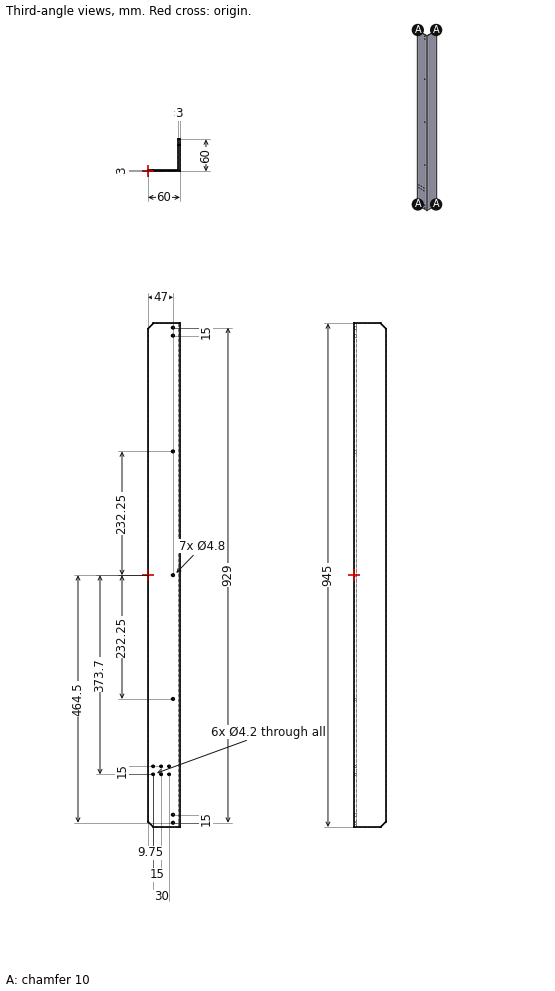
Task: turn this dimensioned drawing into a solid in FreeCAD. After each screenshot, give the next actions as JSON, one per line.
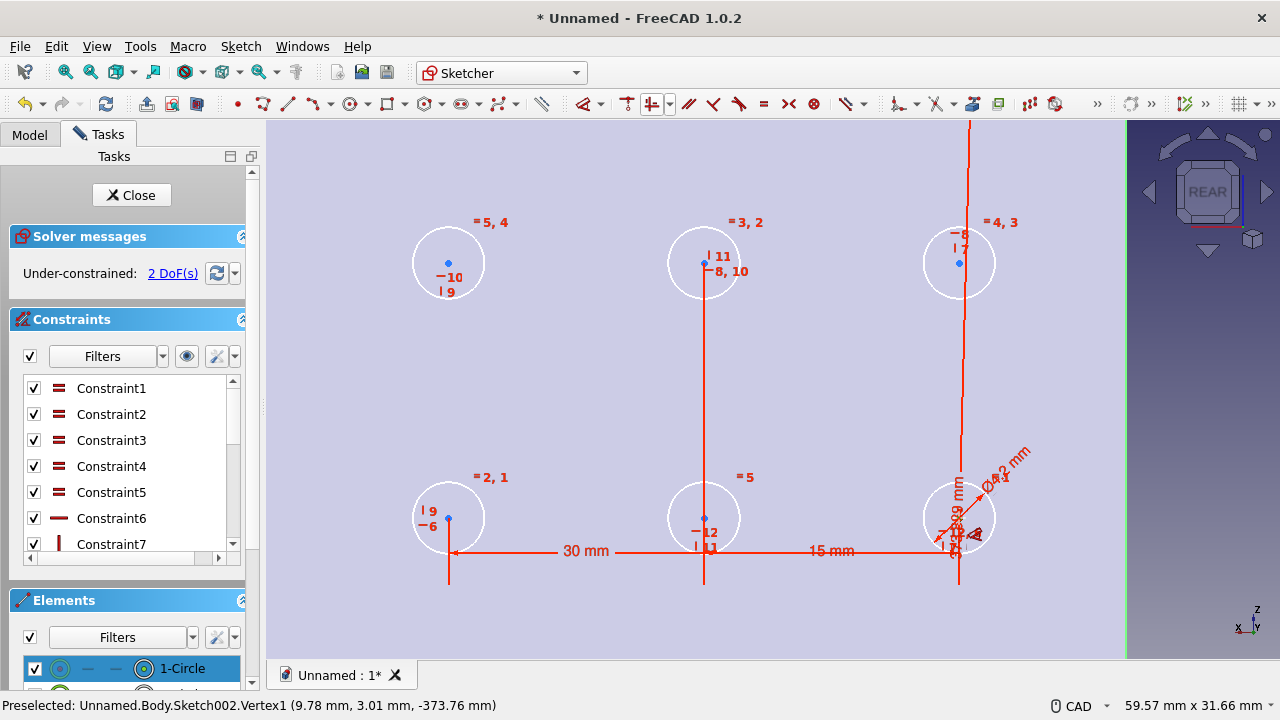
{"action": "left_click", "coordinate": [704, 263]}
{"action": "left_click", "coordinate": [993, 390]}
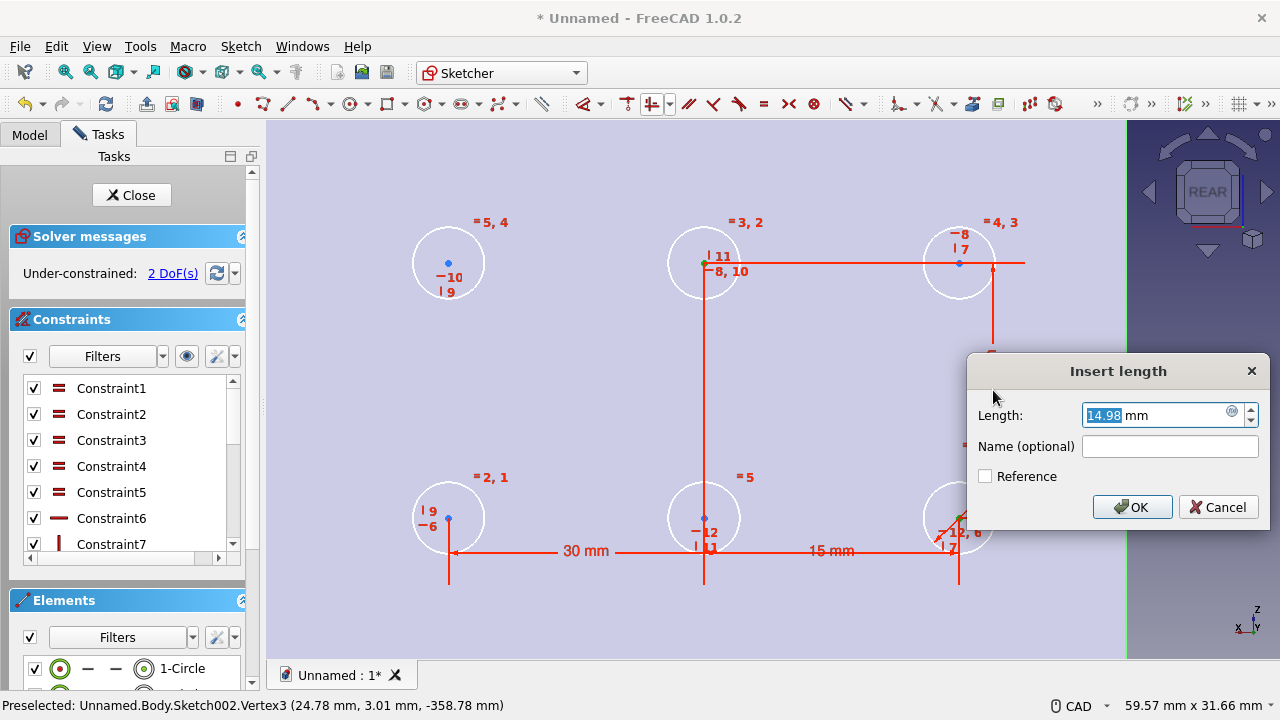
{"action": "type", "text": "15"}
{"action": "key", "text": "Return"}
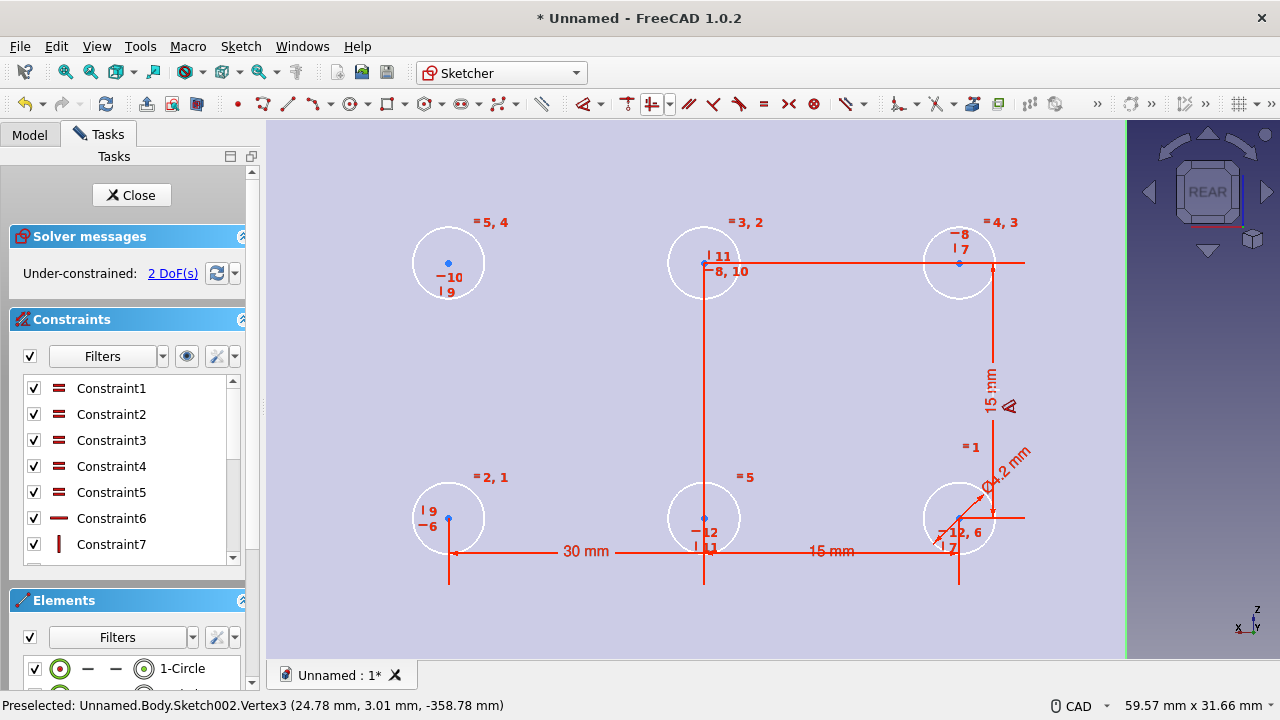
{"action": "left_click", "coordinate": [959, 518]}
{"action": "left_click", "coordinate": [1037, 552]}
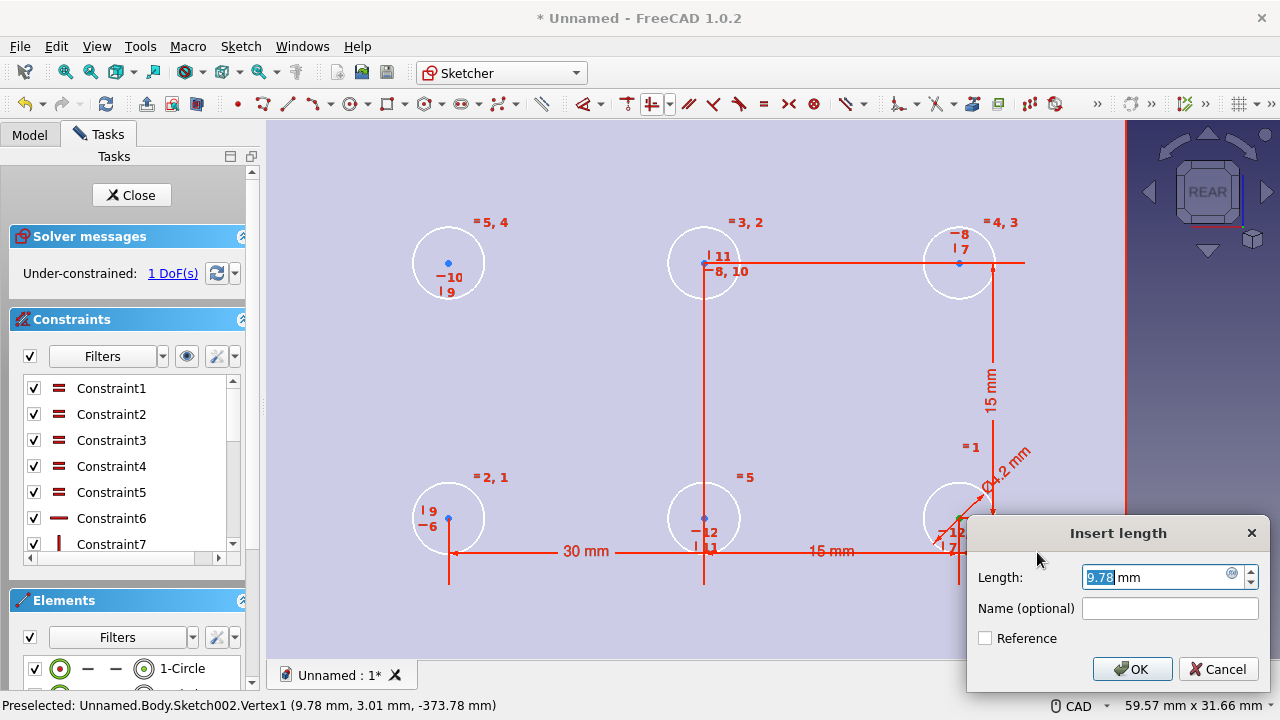
{"action": "type", "text": "9.75"}
{"action": "key", "text": "Return"}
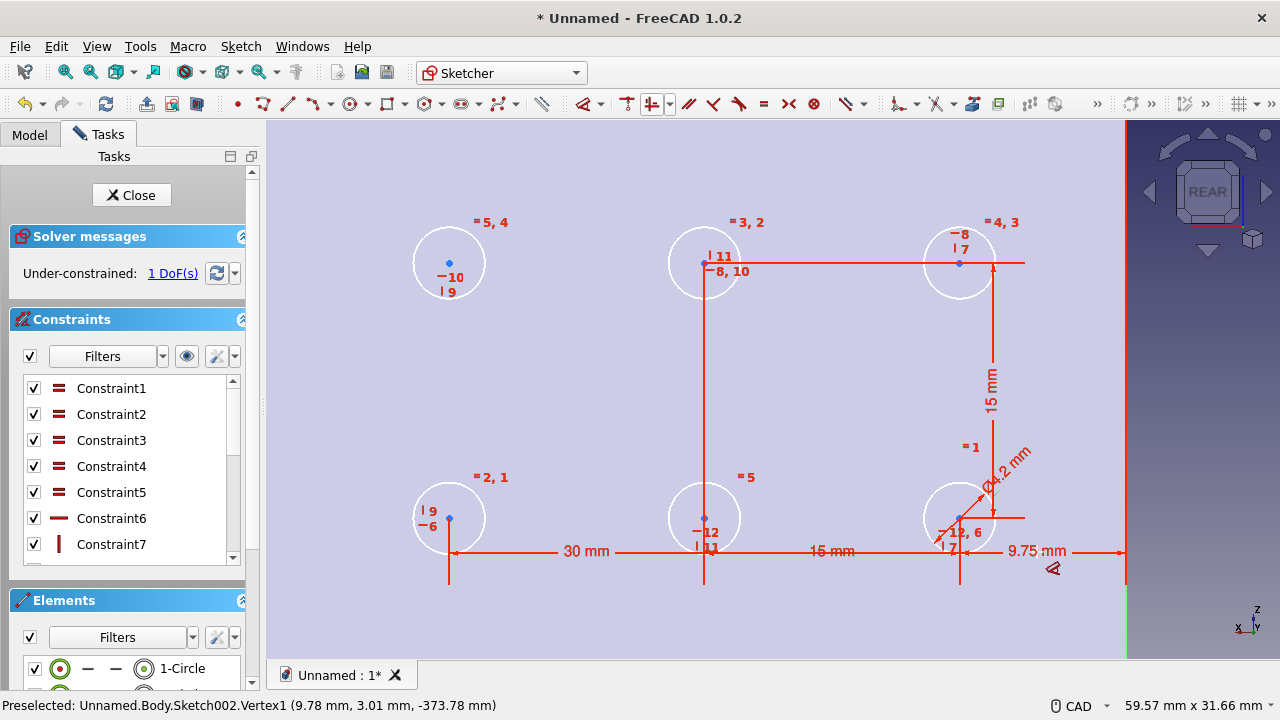
{"action": "left_click", "coordinate": [960, 518]}
{"action": "left_click", "coordinate": [926, 333]}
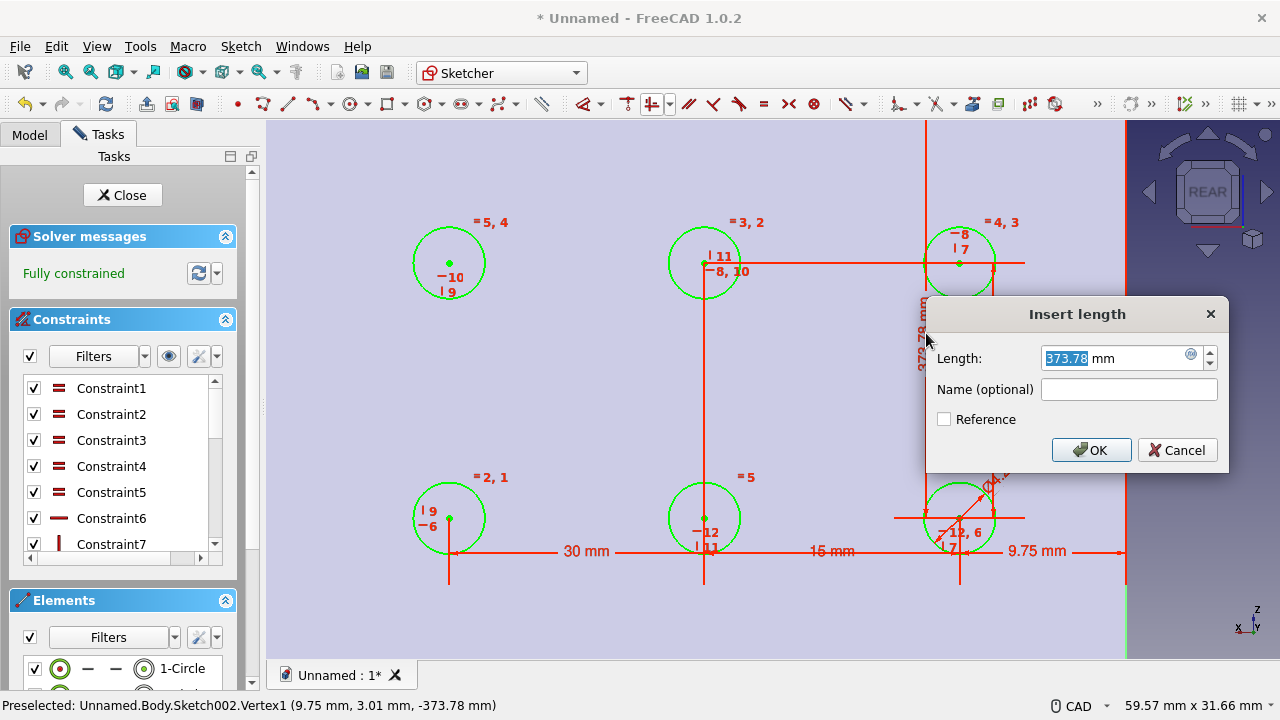
{"action": "type", "text": "373.7"}
{"action": "key", "text": "Return"}
{"action": "key", "text": "Escape"}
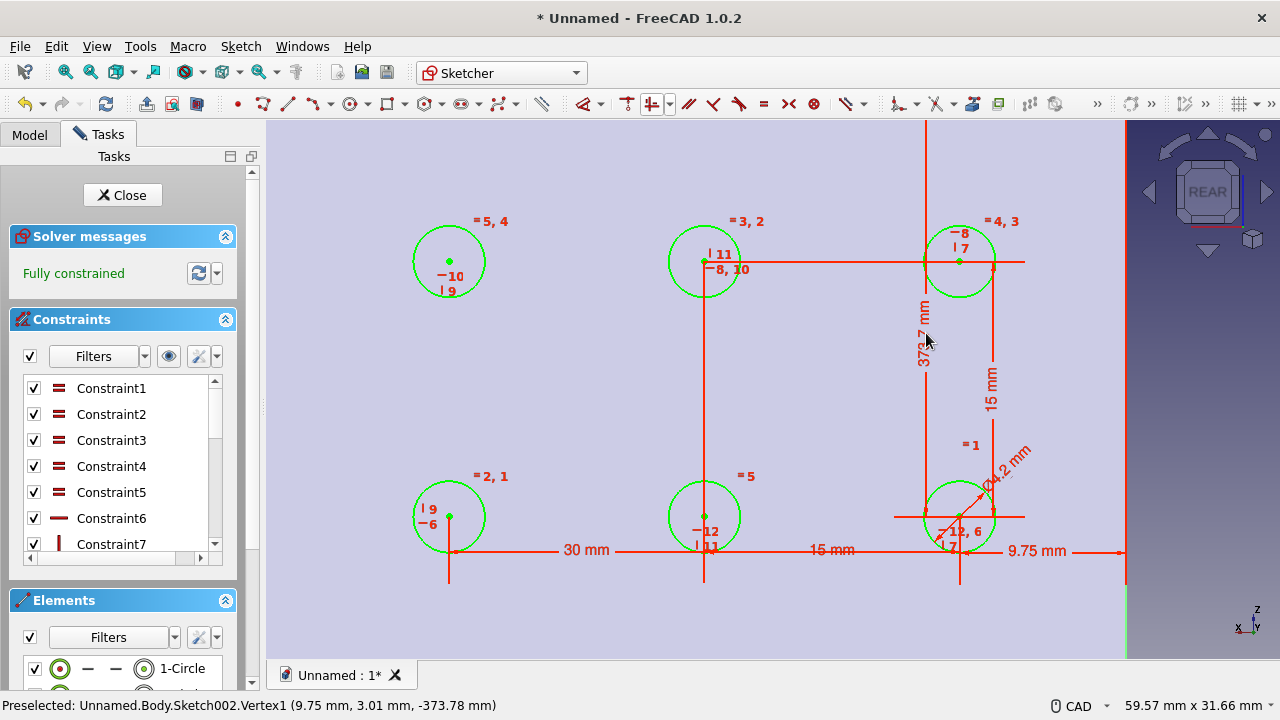
{"action": "left_click", "coordinate": [123, 195]}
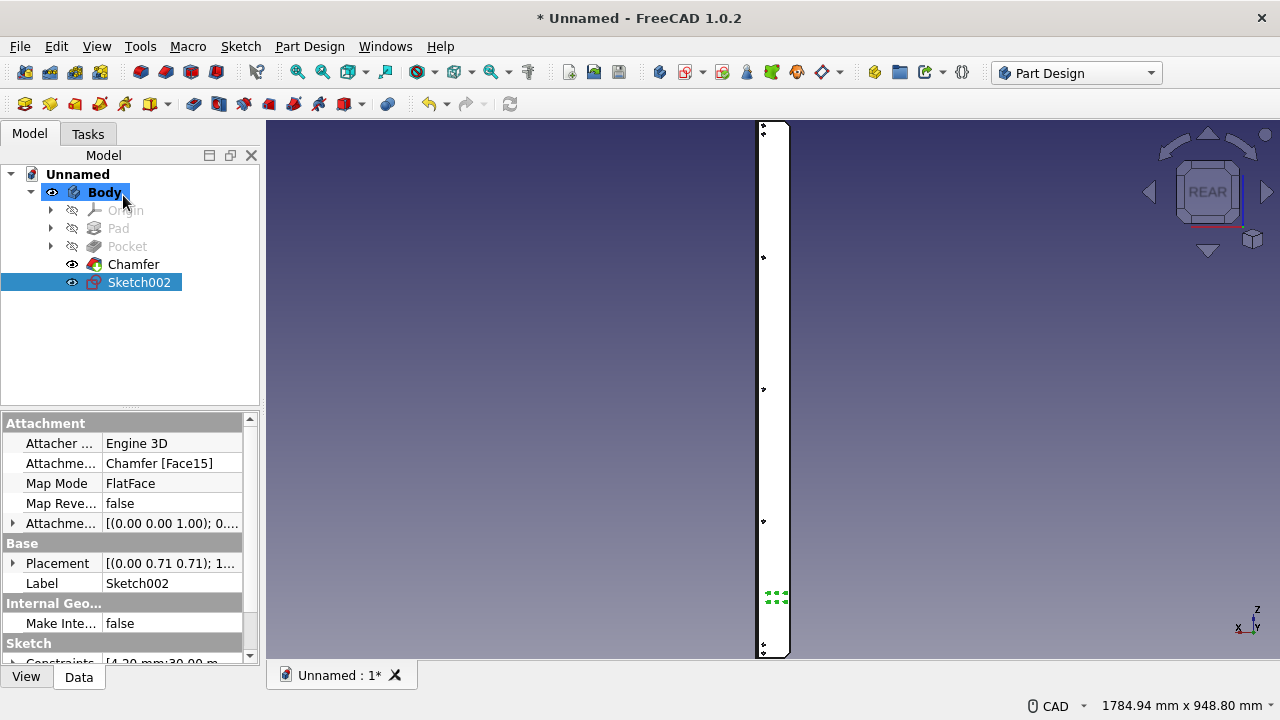
{"action": "left_click", "coordinate": [219, 104]}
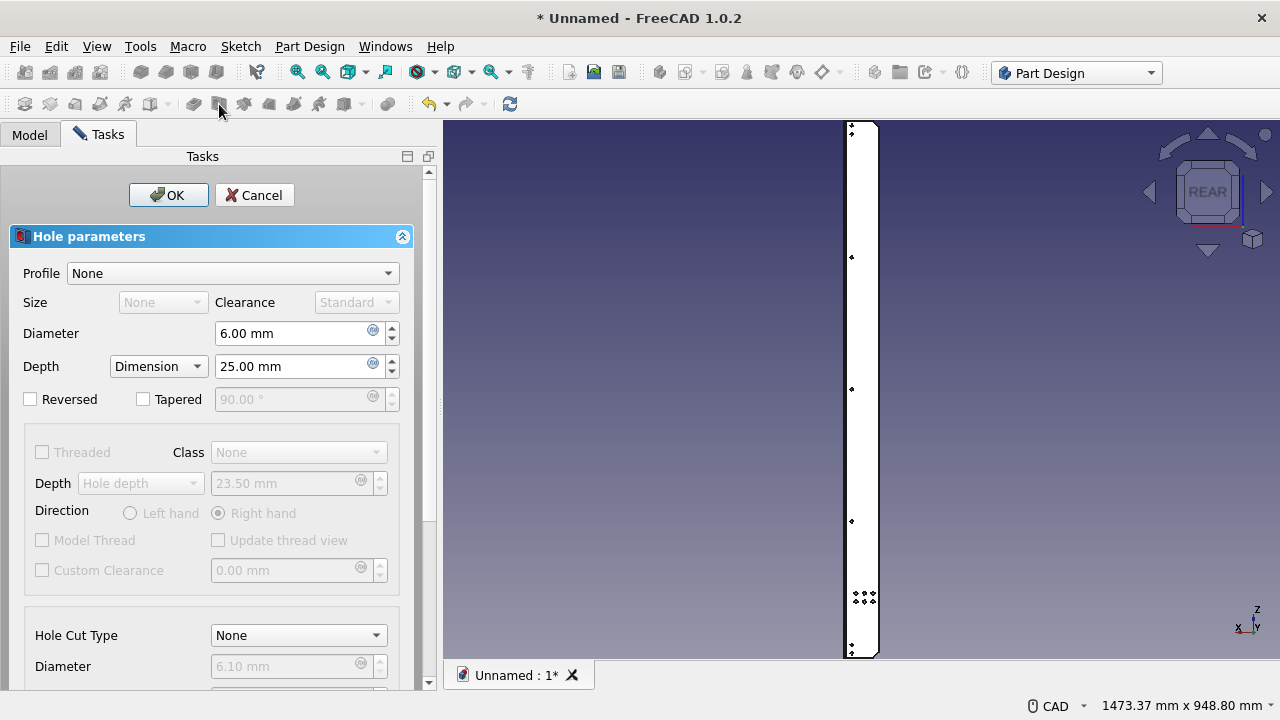
{"action": "triple_click", "coordinate": [300, 334]}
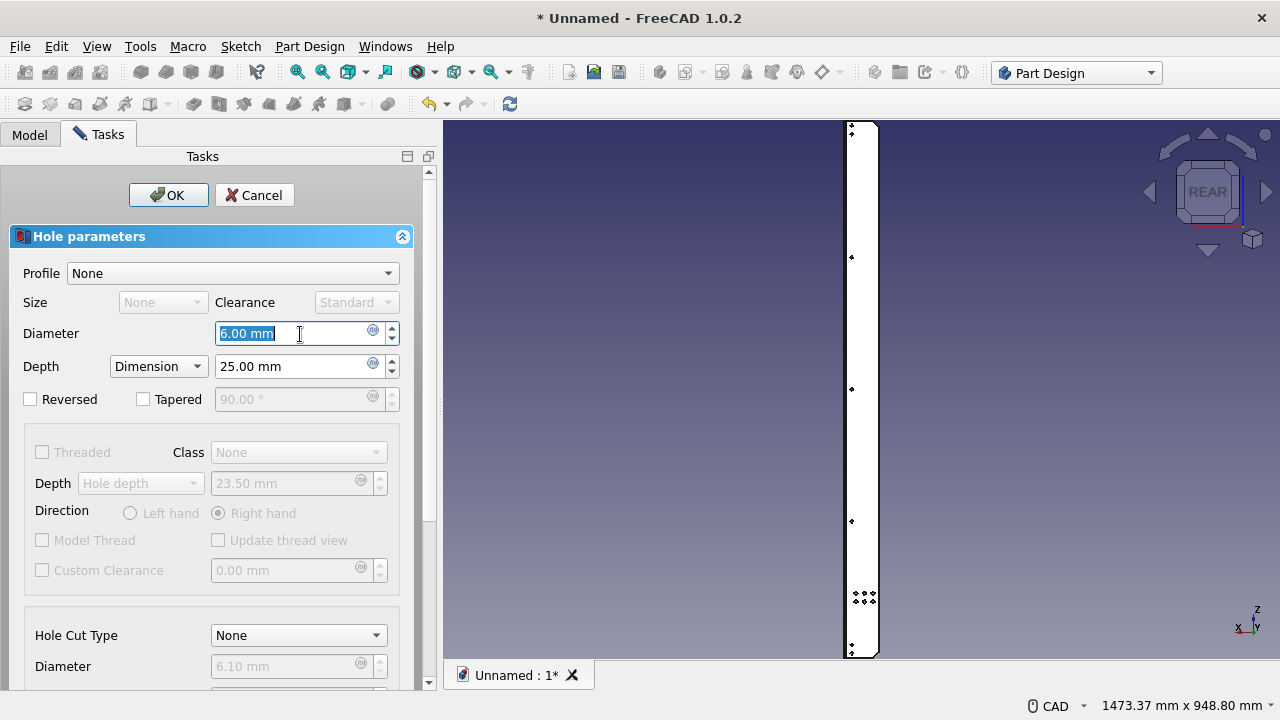
{"action": "type", "text": "4.2"}
{"action": "key", "text": "Tab"}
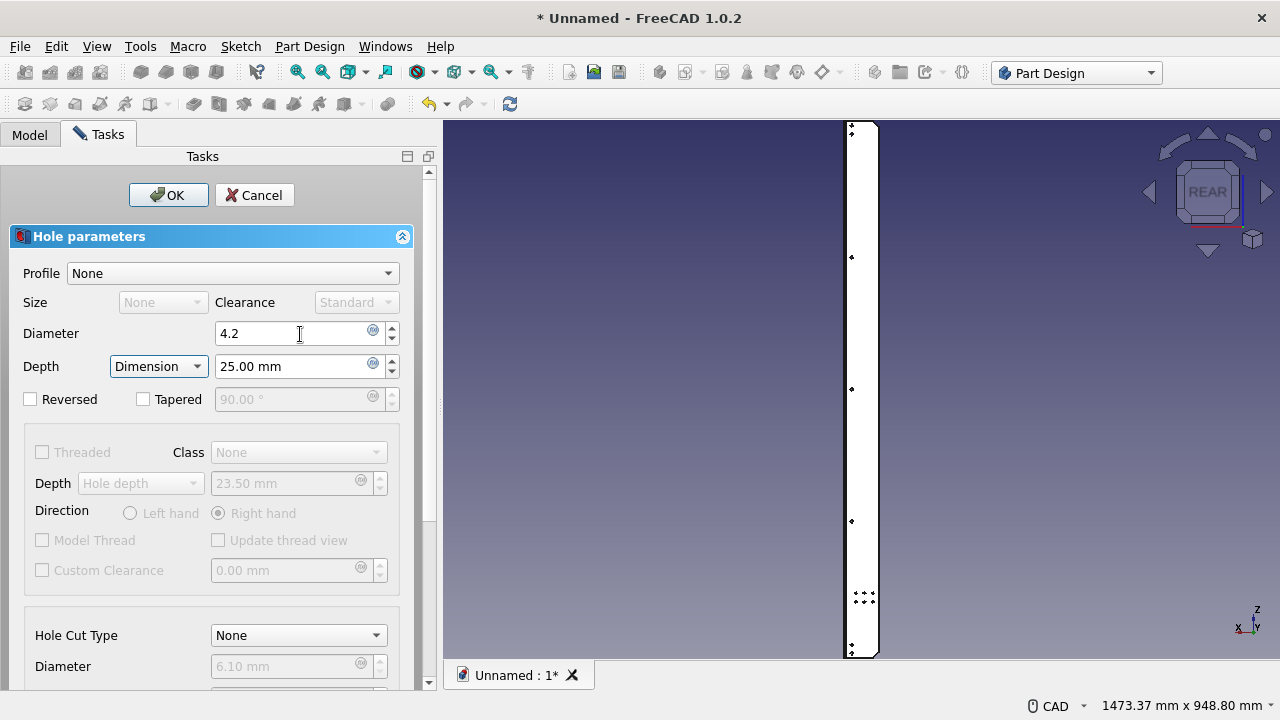
{"action": "left_click", "coordinate": [160, 366]}